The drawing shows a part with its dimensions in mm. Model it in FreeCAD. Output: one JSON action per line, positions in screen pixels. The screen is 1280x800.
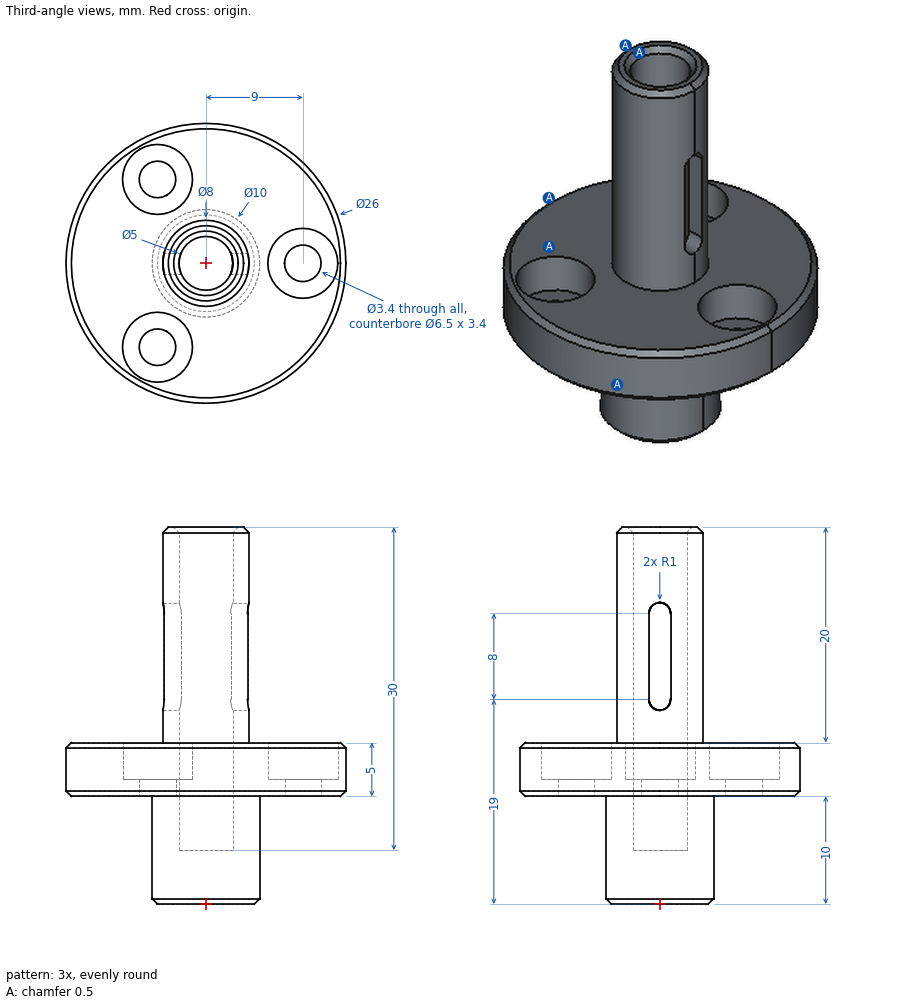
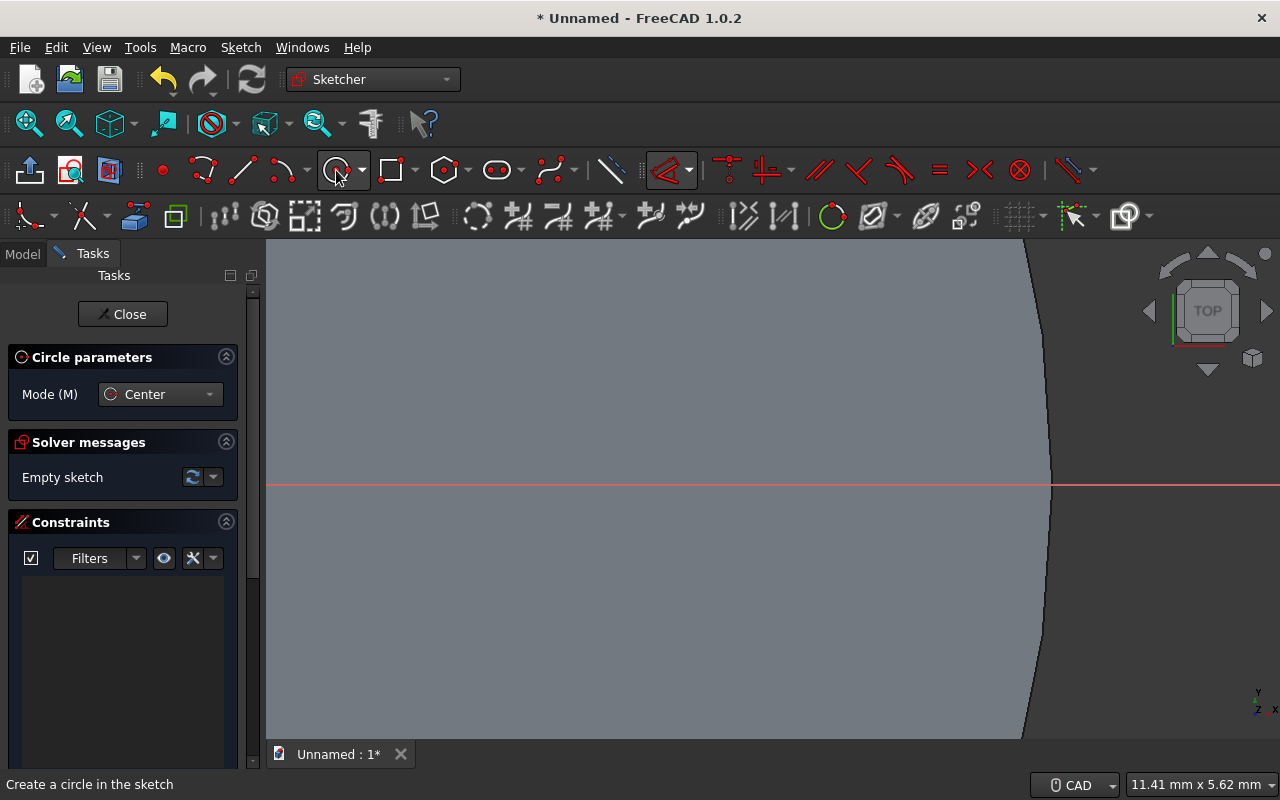
{"action": "left_click", "coordinate": [697, 485]}
{"action": "left_click", "coordinate": [804, 378]}
{"action": "key", "text": "Escape"}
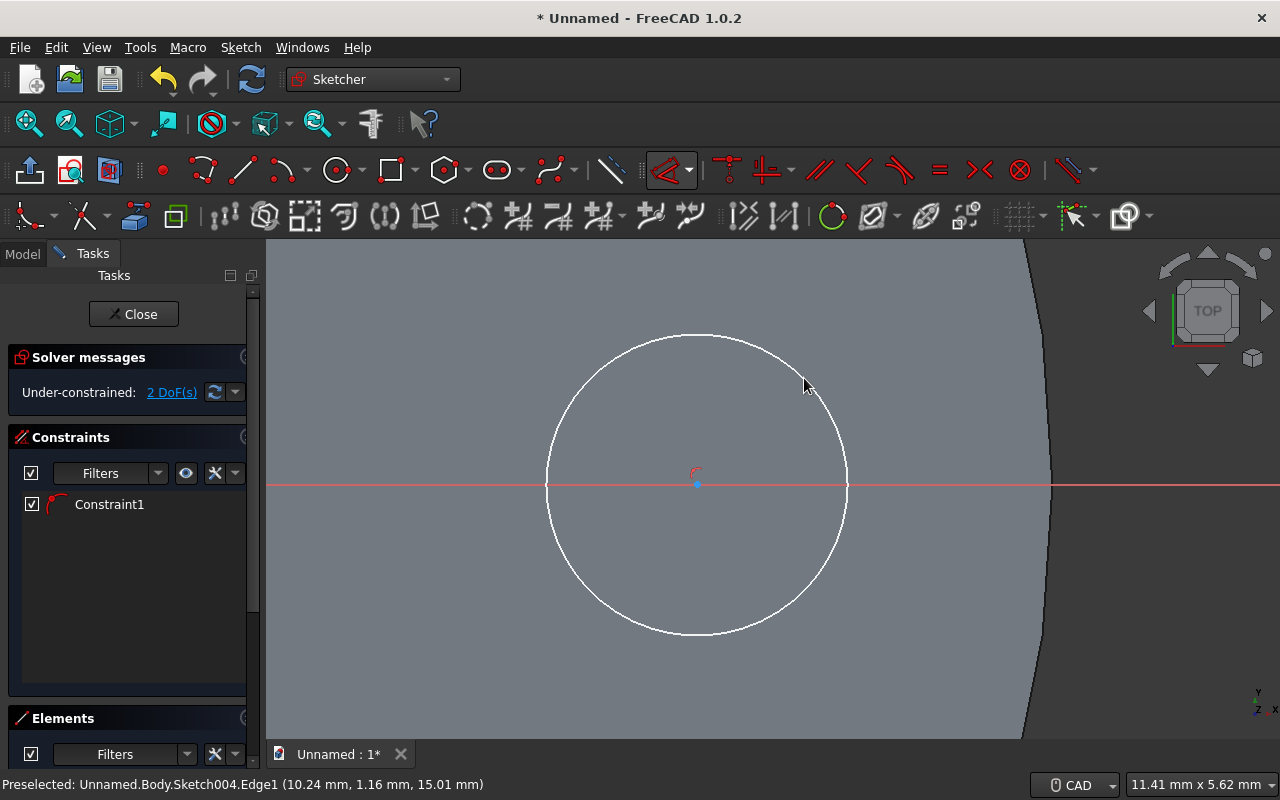
{"action": "left_click", "coordinate": [803, 378]}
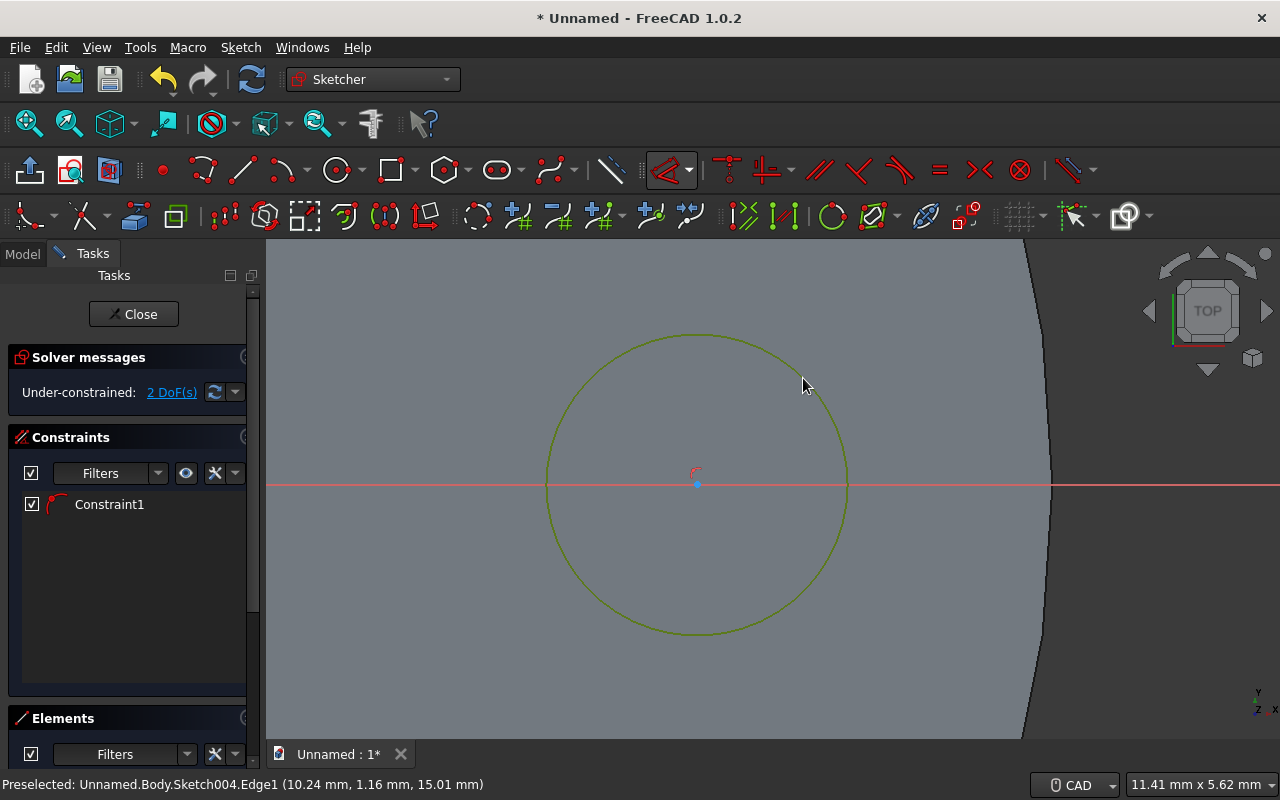
{"action": "left_click", "coordinate": [692, 170]}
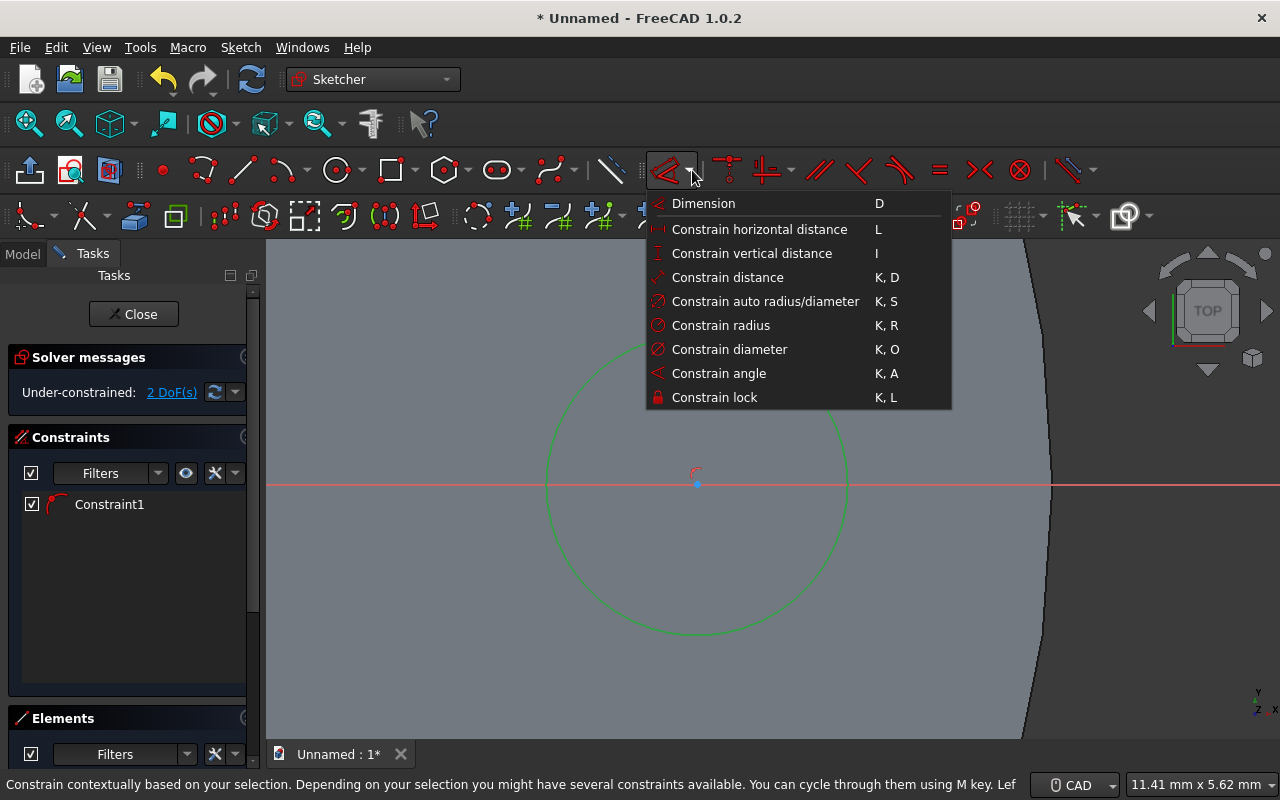
{"action": "left_click", "coordinate": [799, 349]}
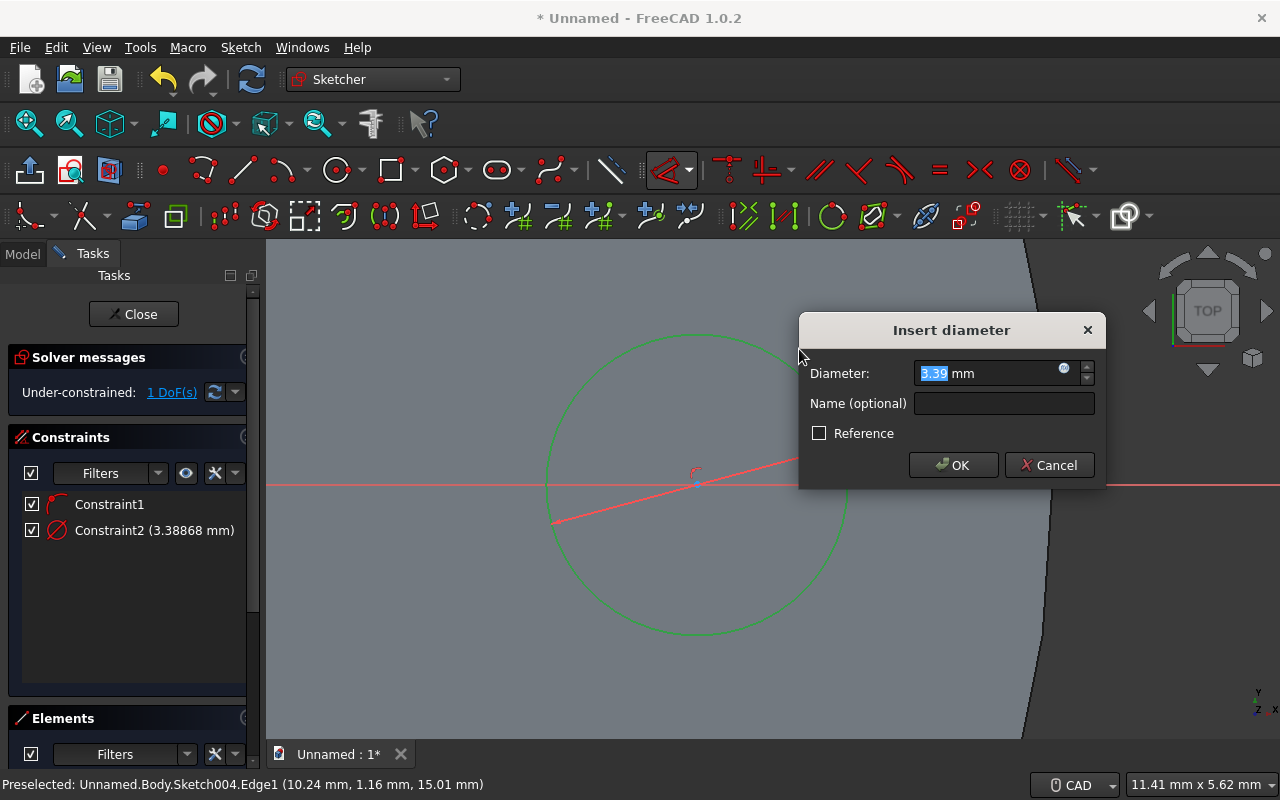
{"action": "type", "text": "3.4"}
{"action": "key", "text": "Return"}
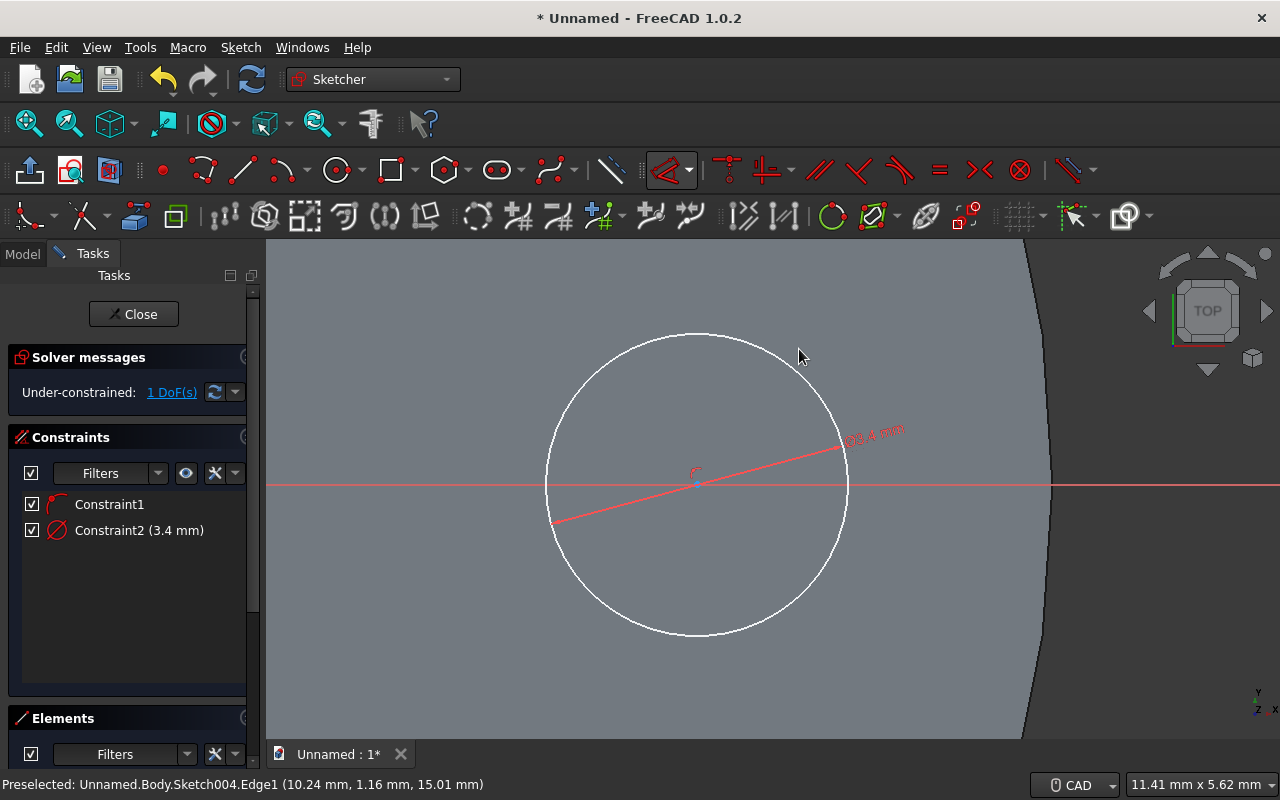
{"action": "left_click", "coordinate": [697, 485]}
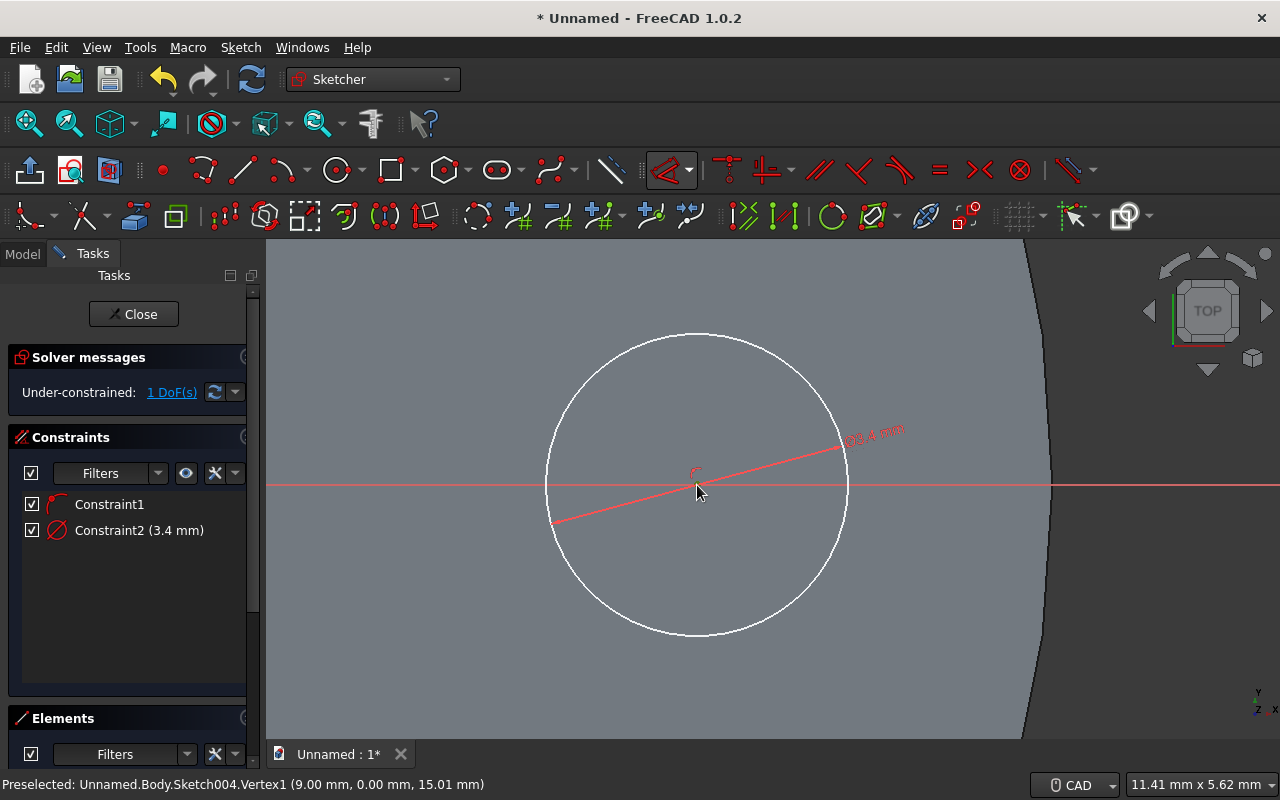
{"action": "key", "text": "l"}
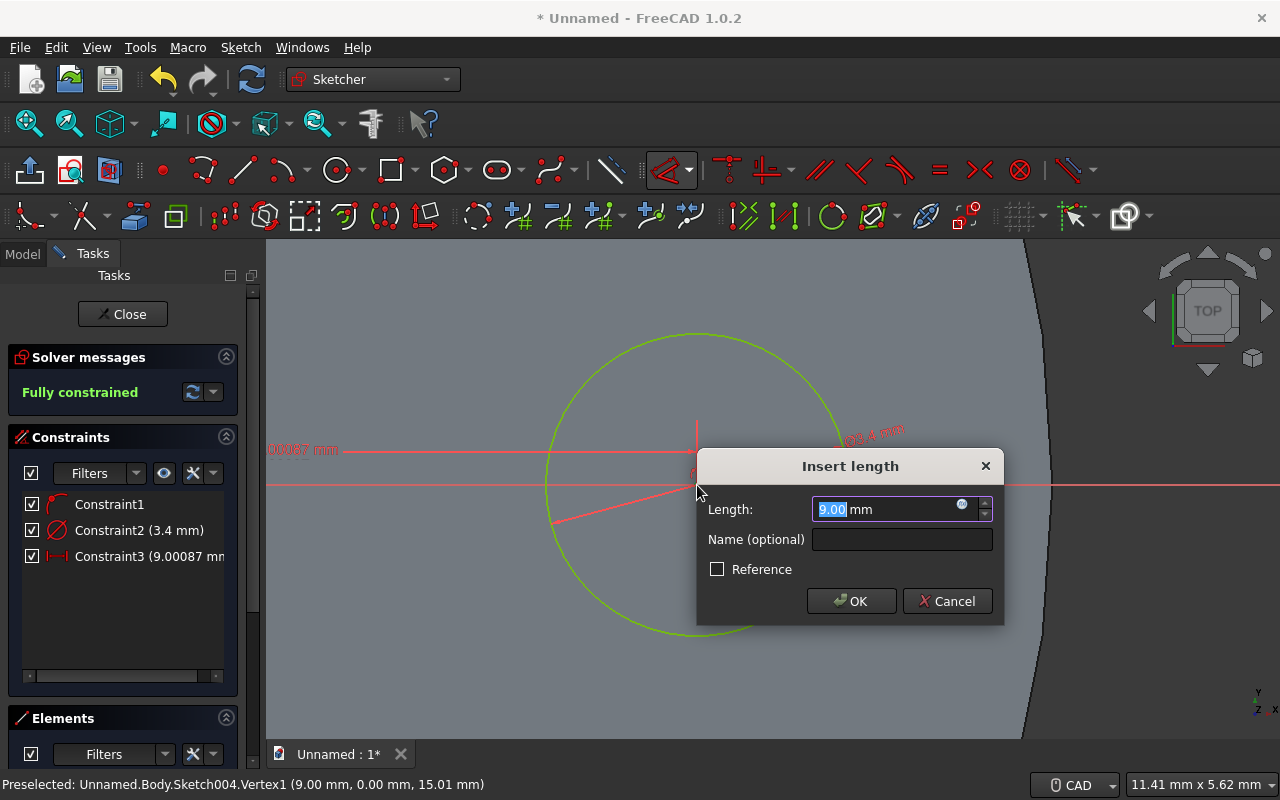
{"action": "type", "text": "9"}
{"action": "key", "text": "Return"}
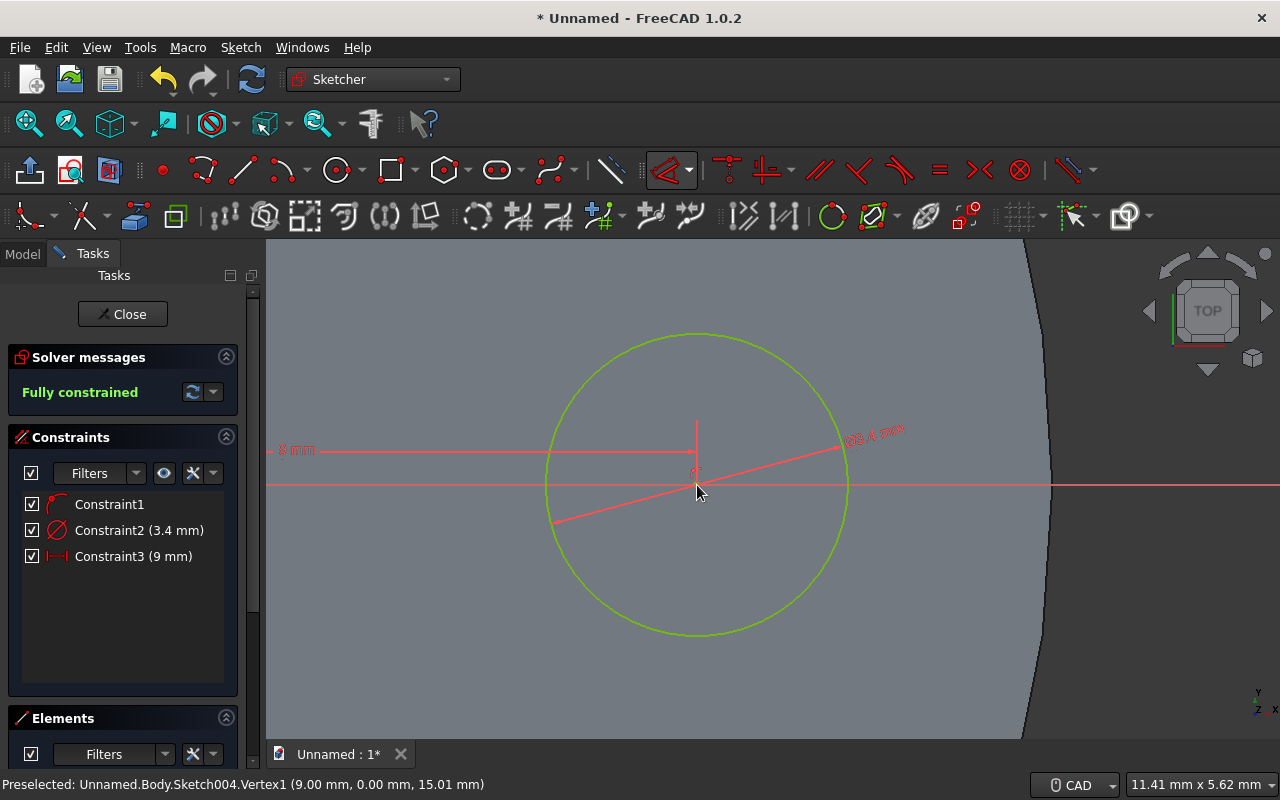
{"action": "left_click", "coordinate": [123, 314]}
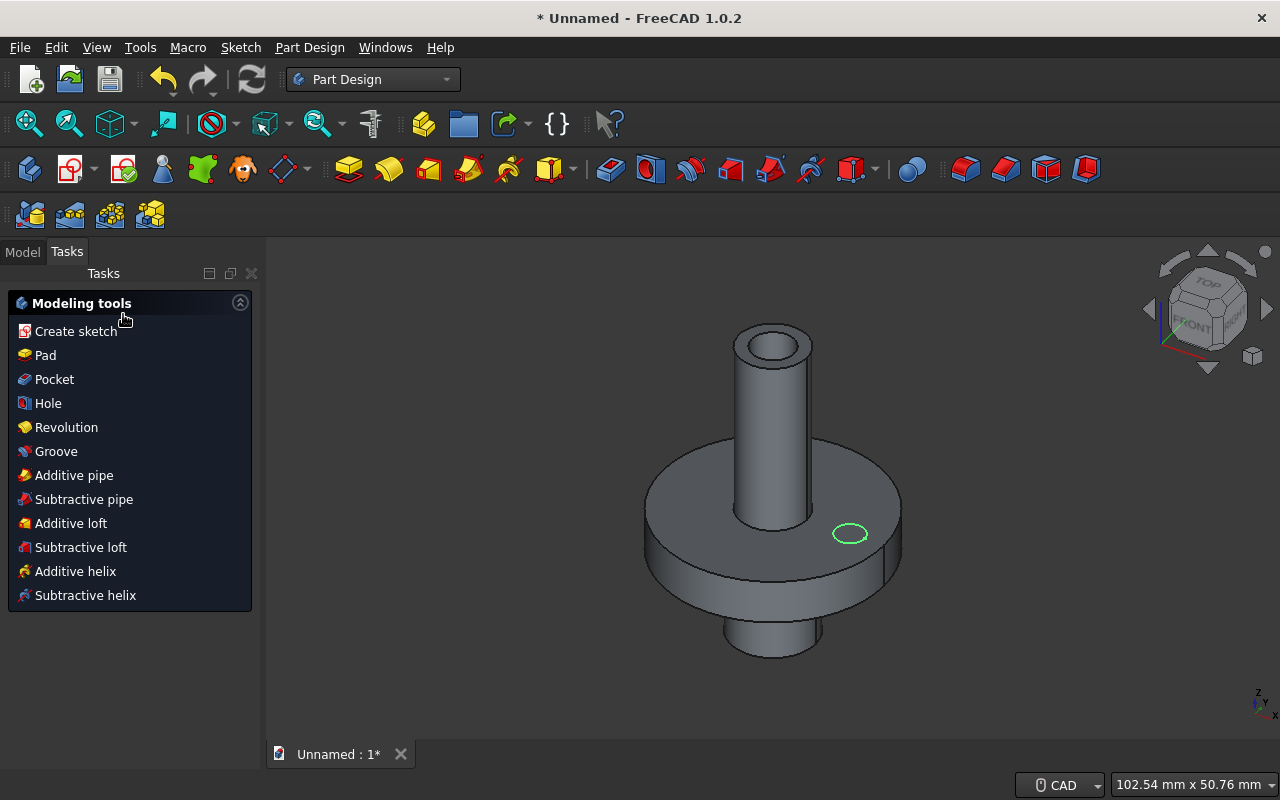
{"action": "left_click", "coordinate": [652, 170]}